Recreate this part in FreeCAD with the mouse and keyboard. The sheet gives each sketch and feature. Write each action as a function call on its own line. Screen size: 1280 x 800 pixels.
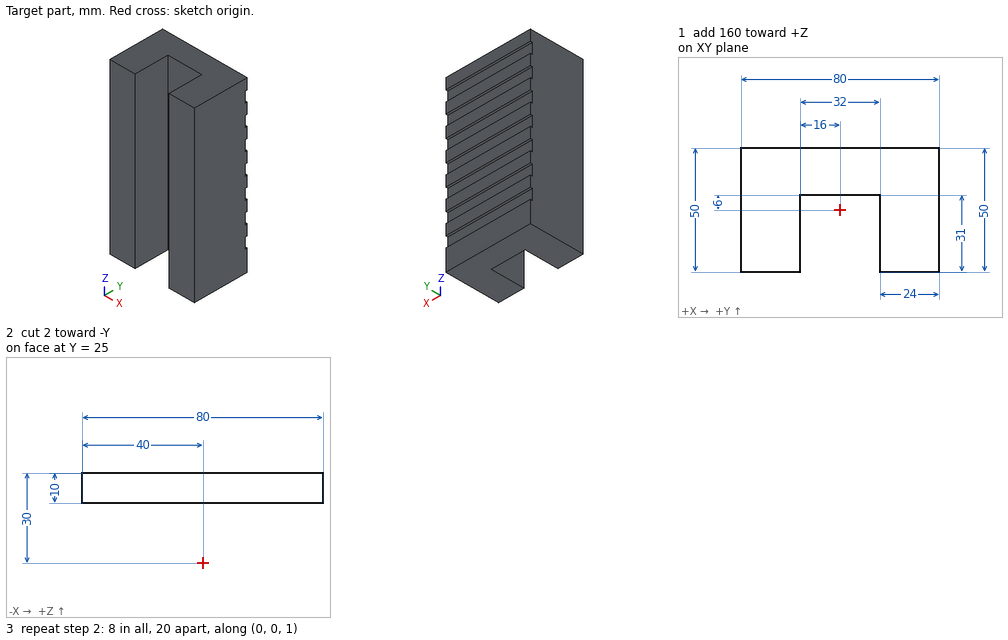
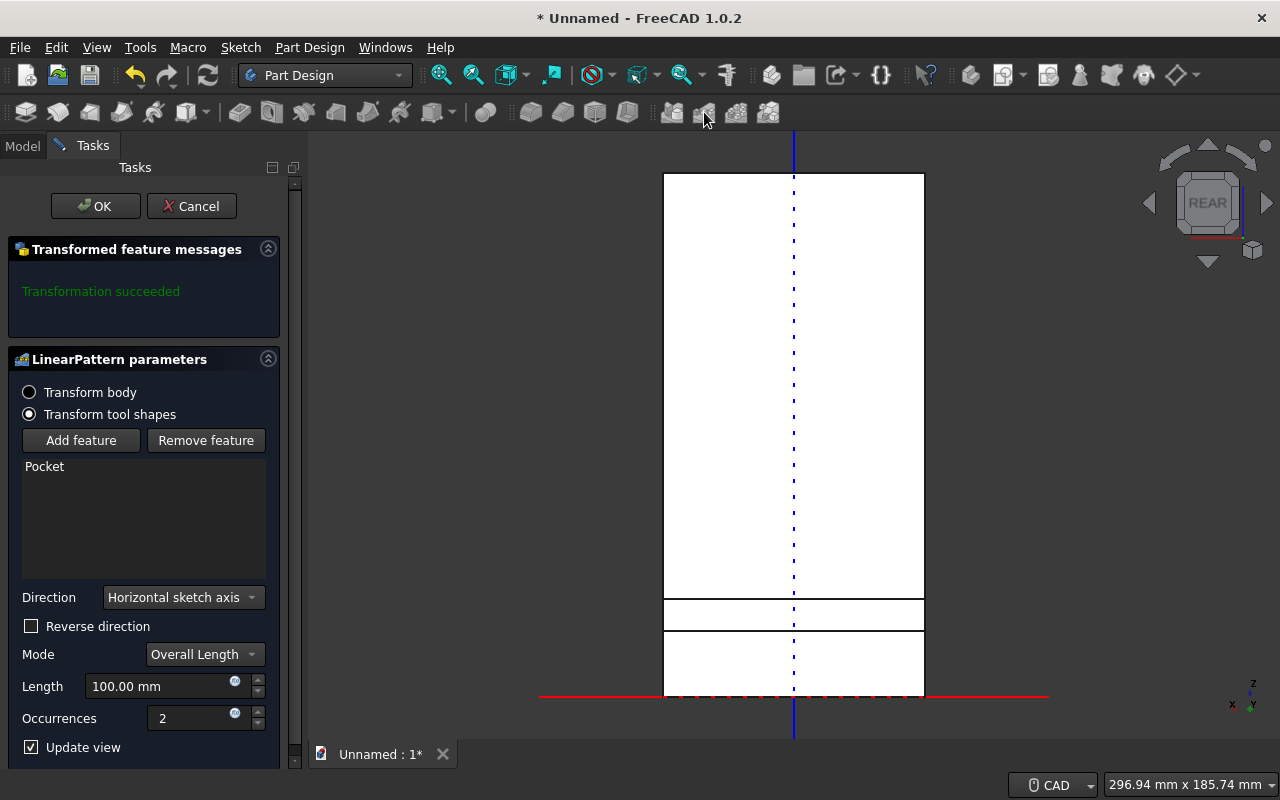
click(184, 598)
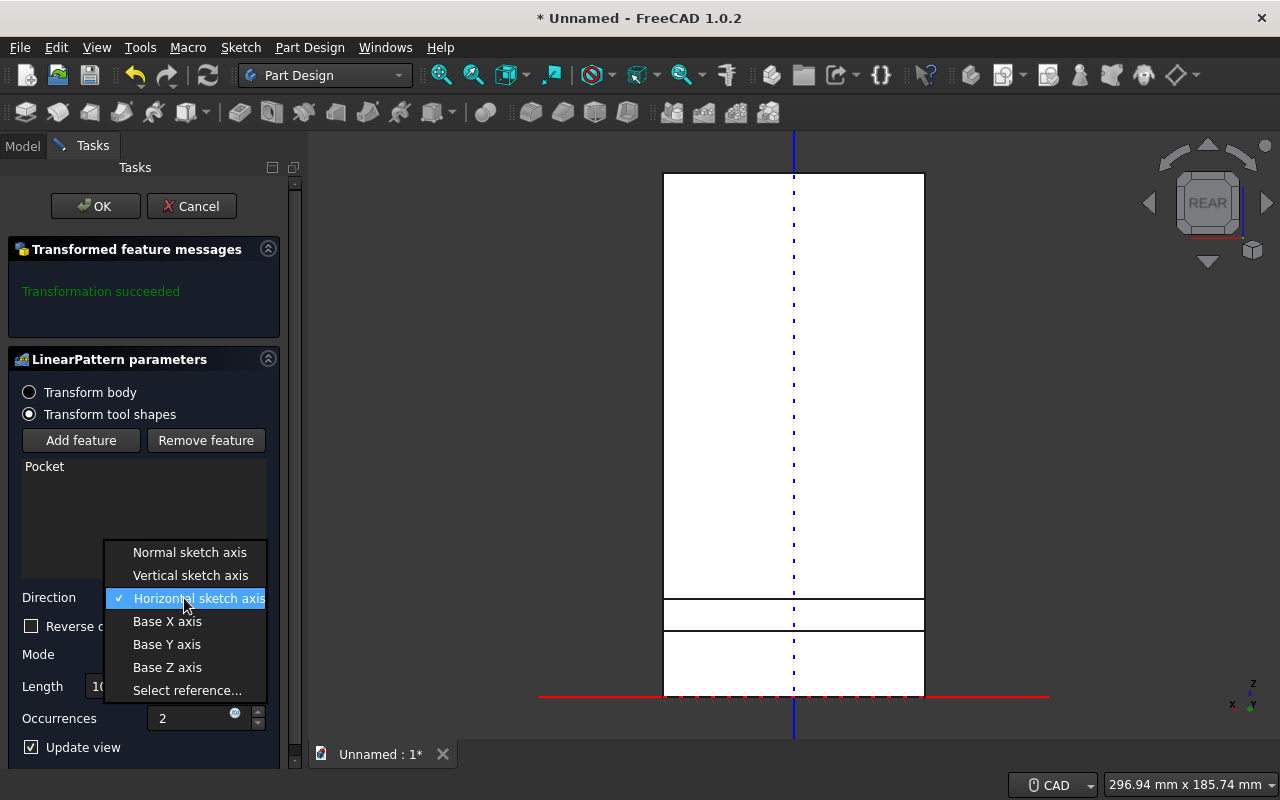
click(184, 668)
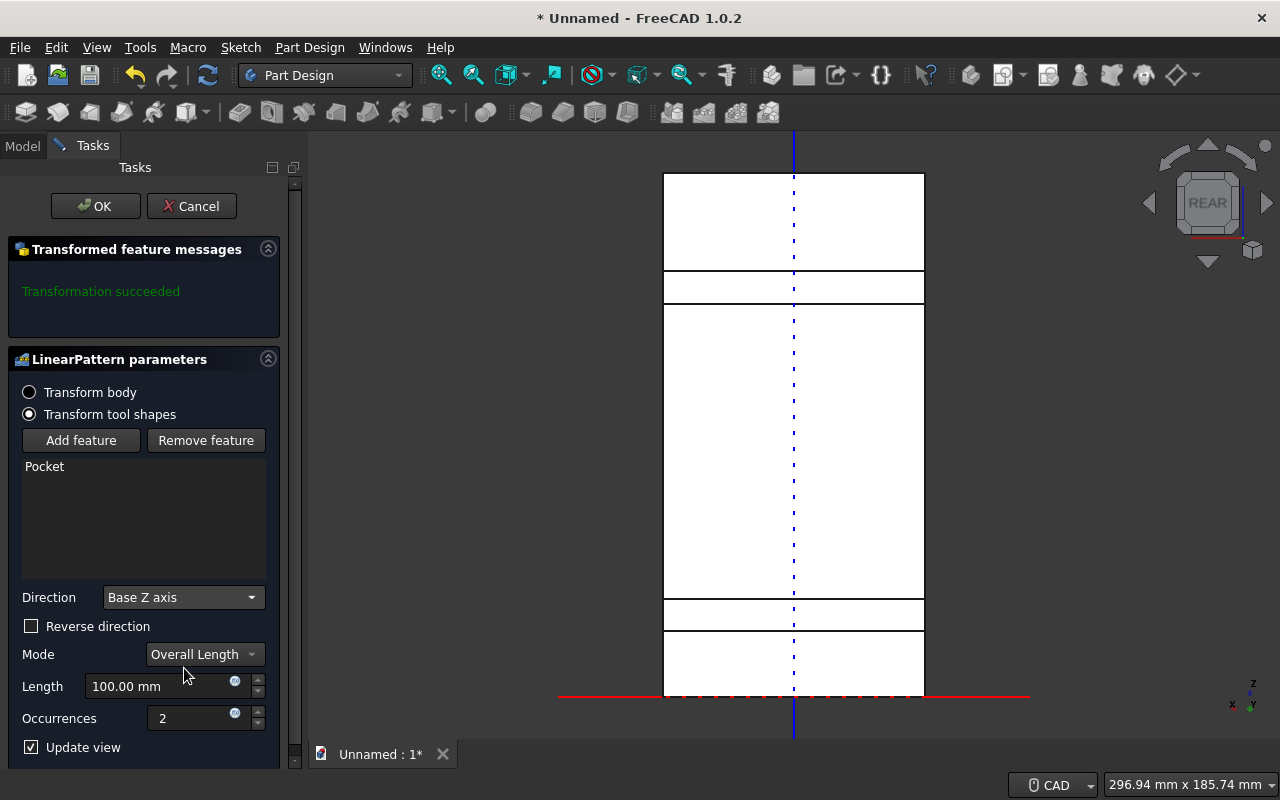
click(206, 654)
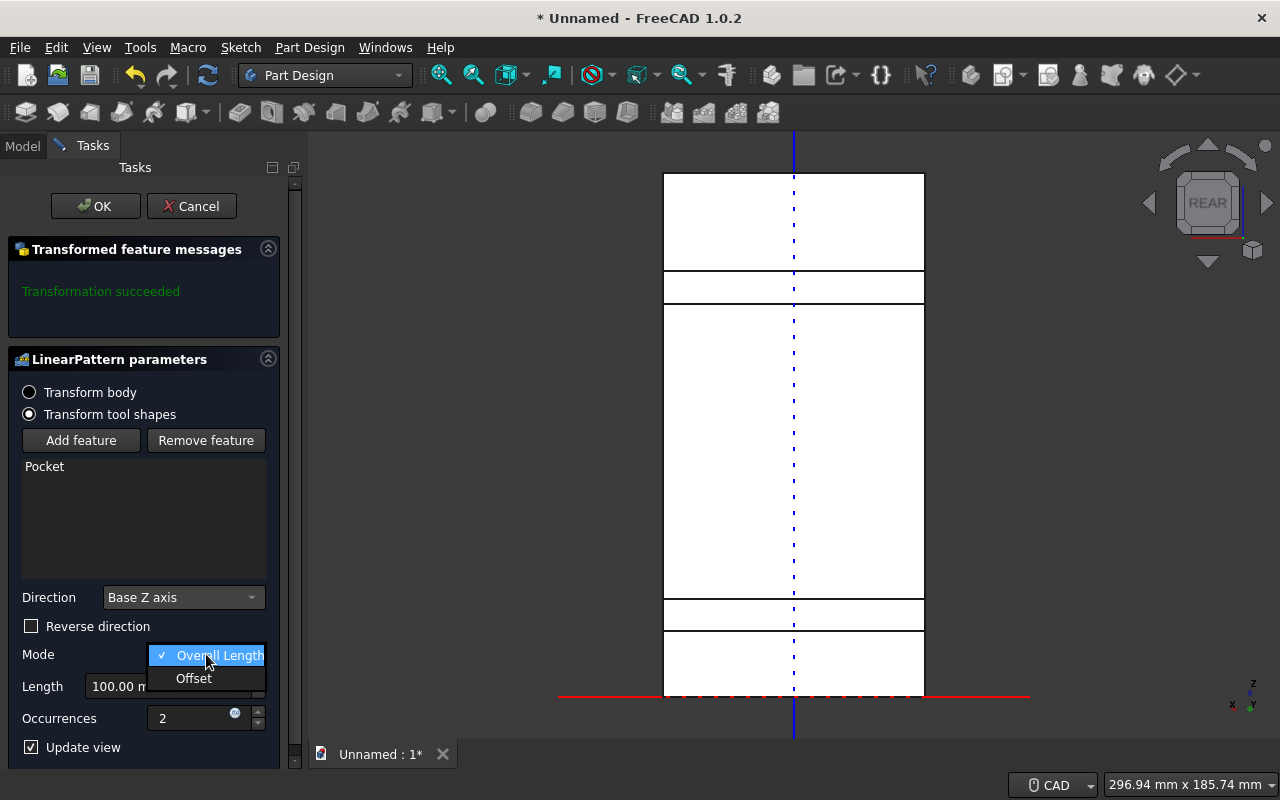
click(206, 678)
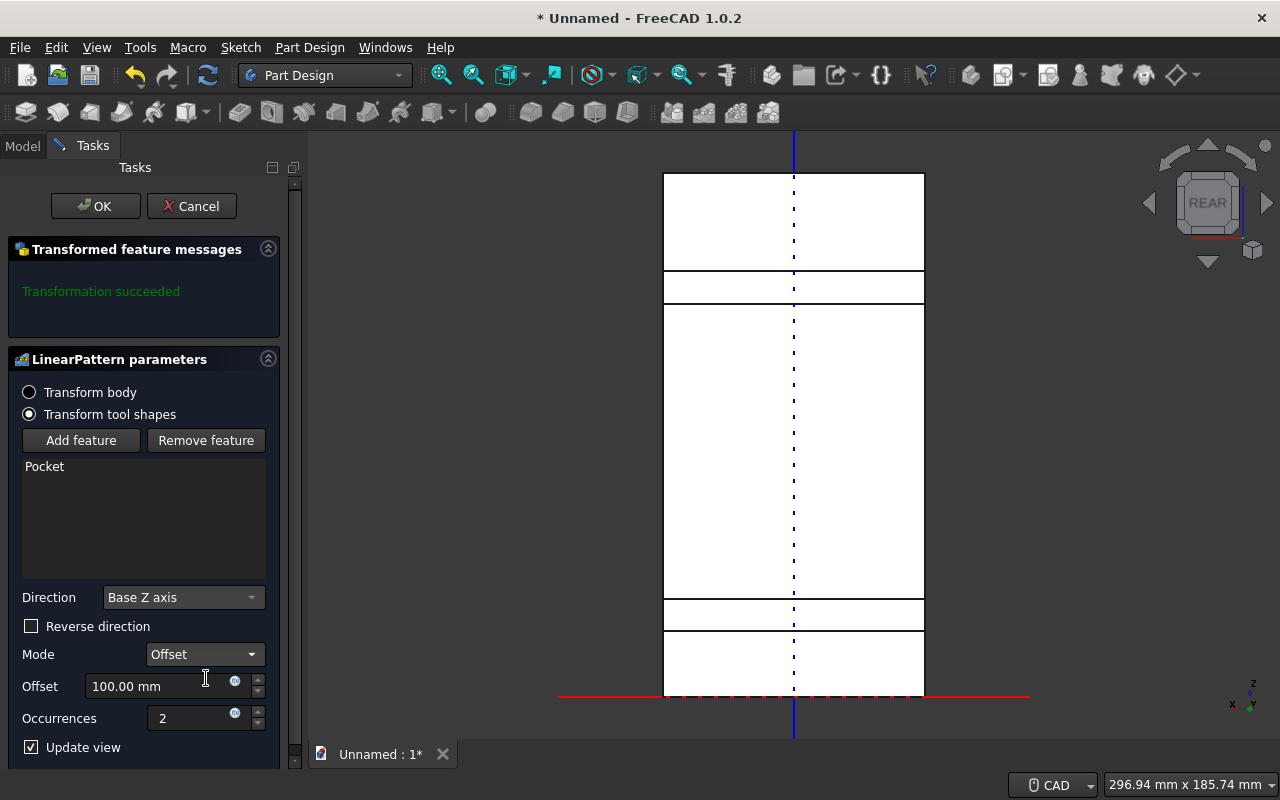
triple_click(168, 686)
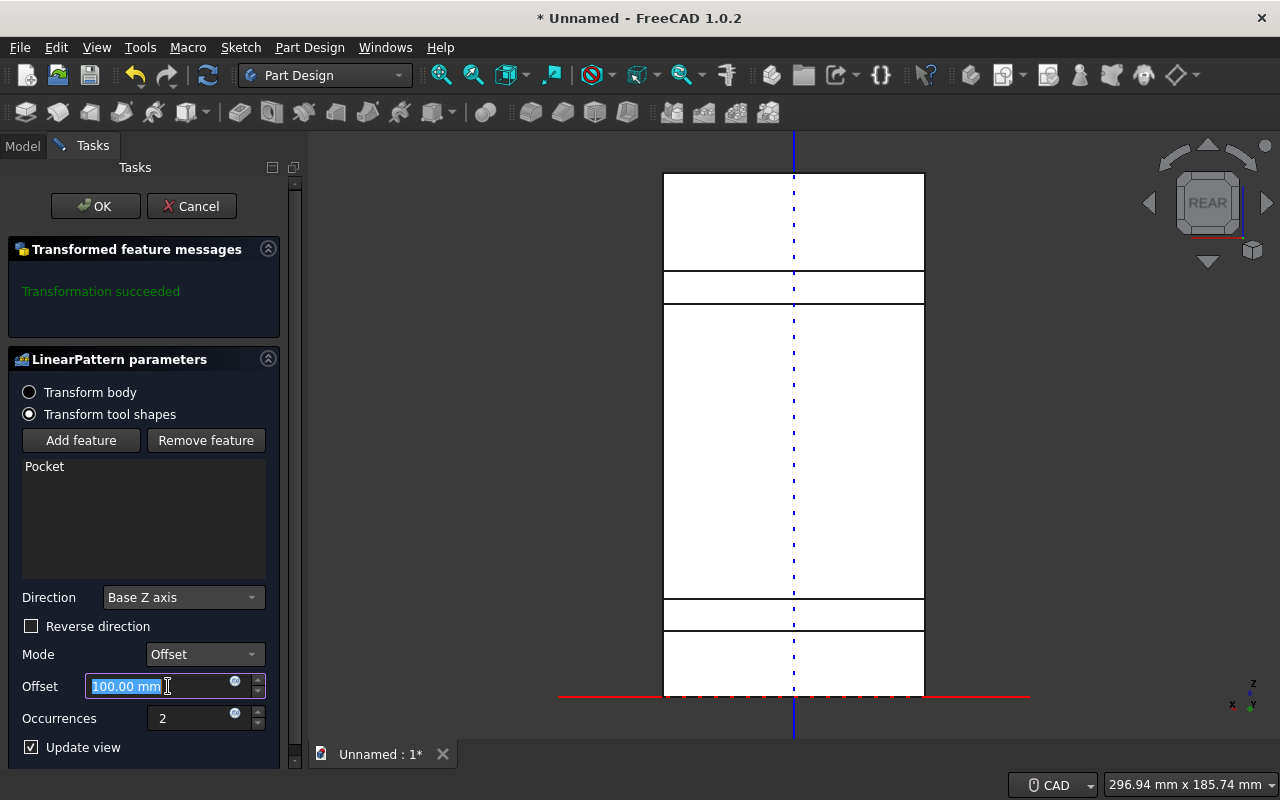
text(20)
key(Tab)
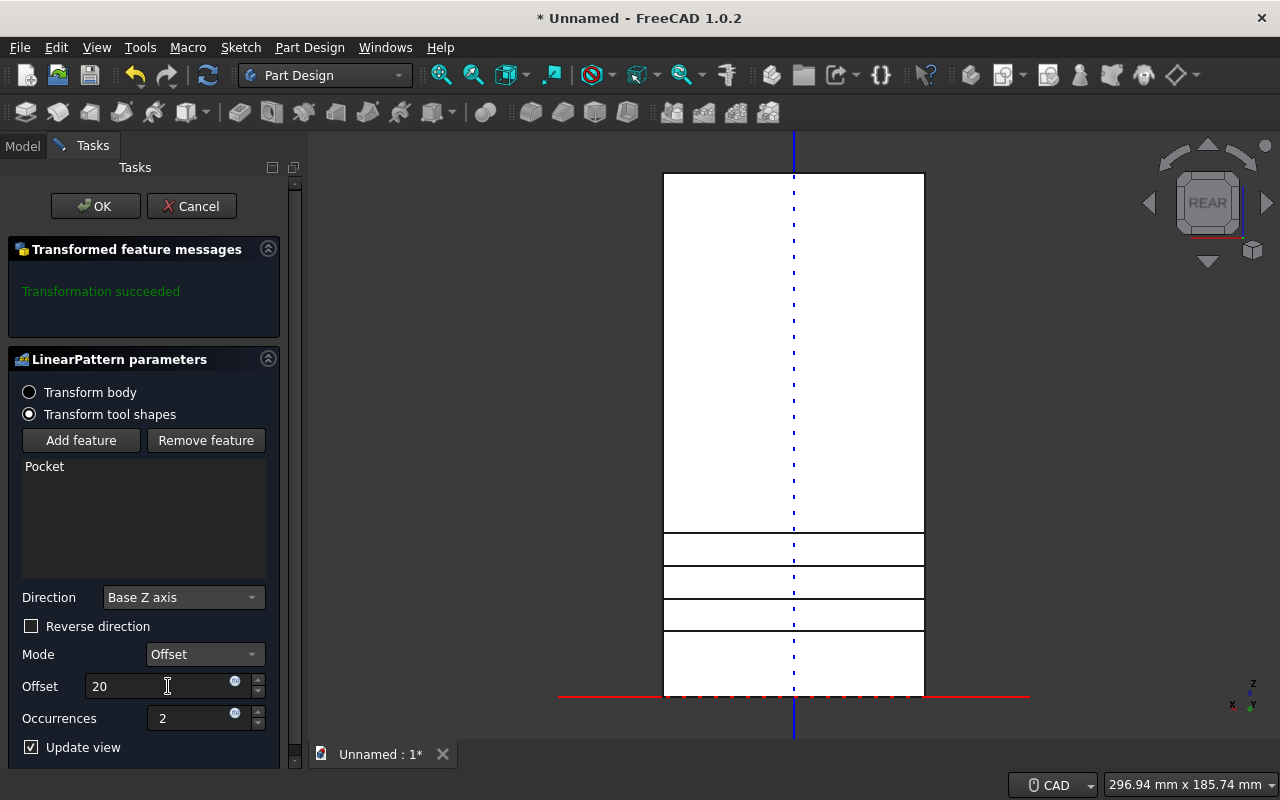
triple_click(198, 718)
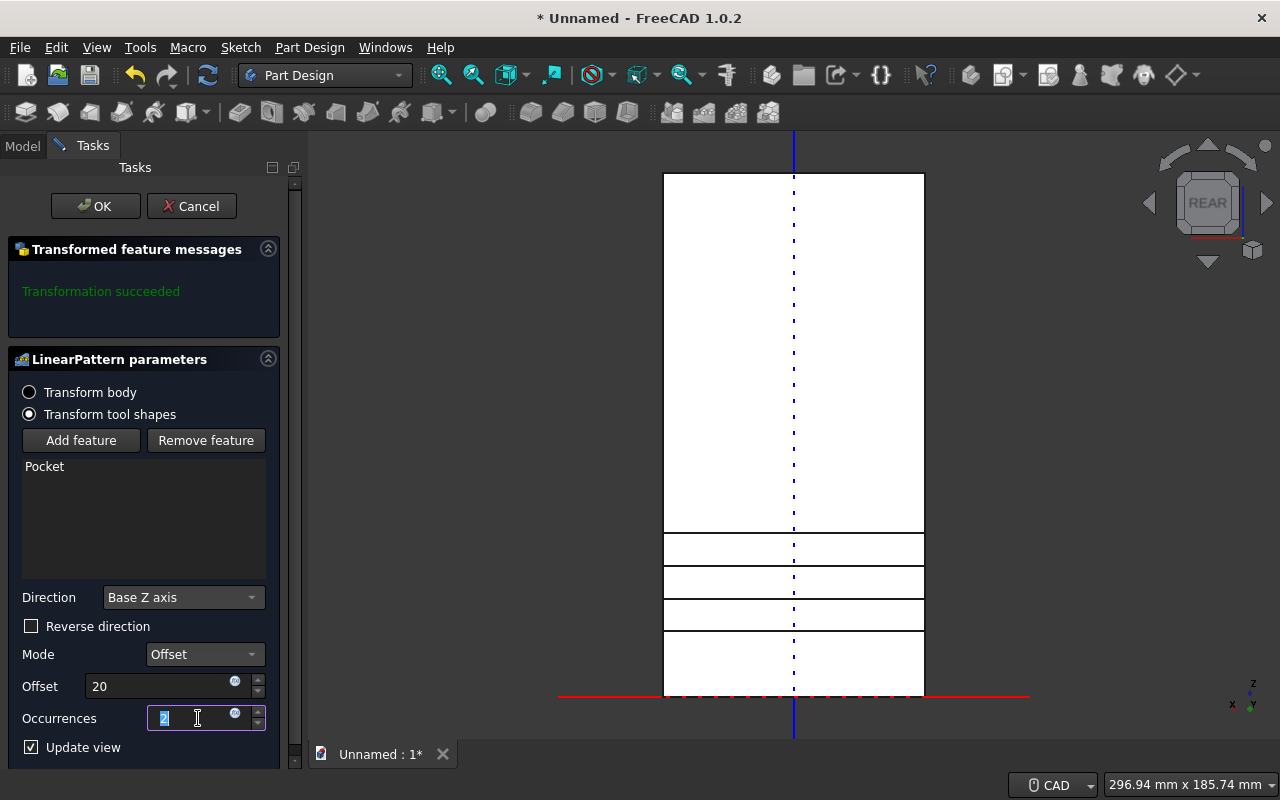
text(8)
key(Tab)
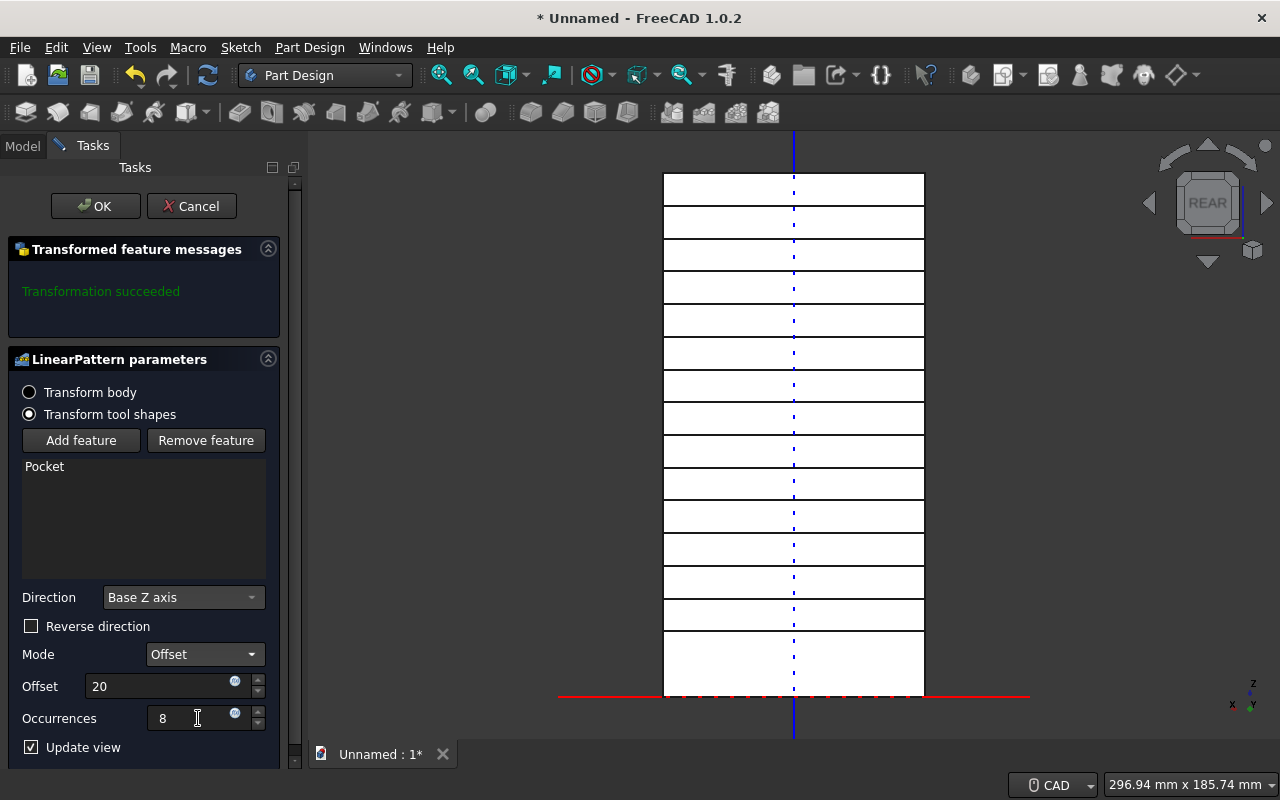
click(96, 206)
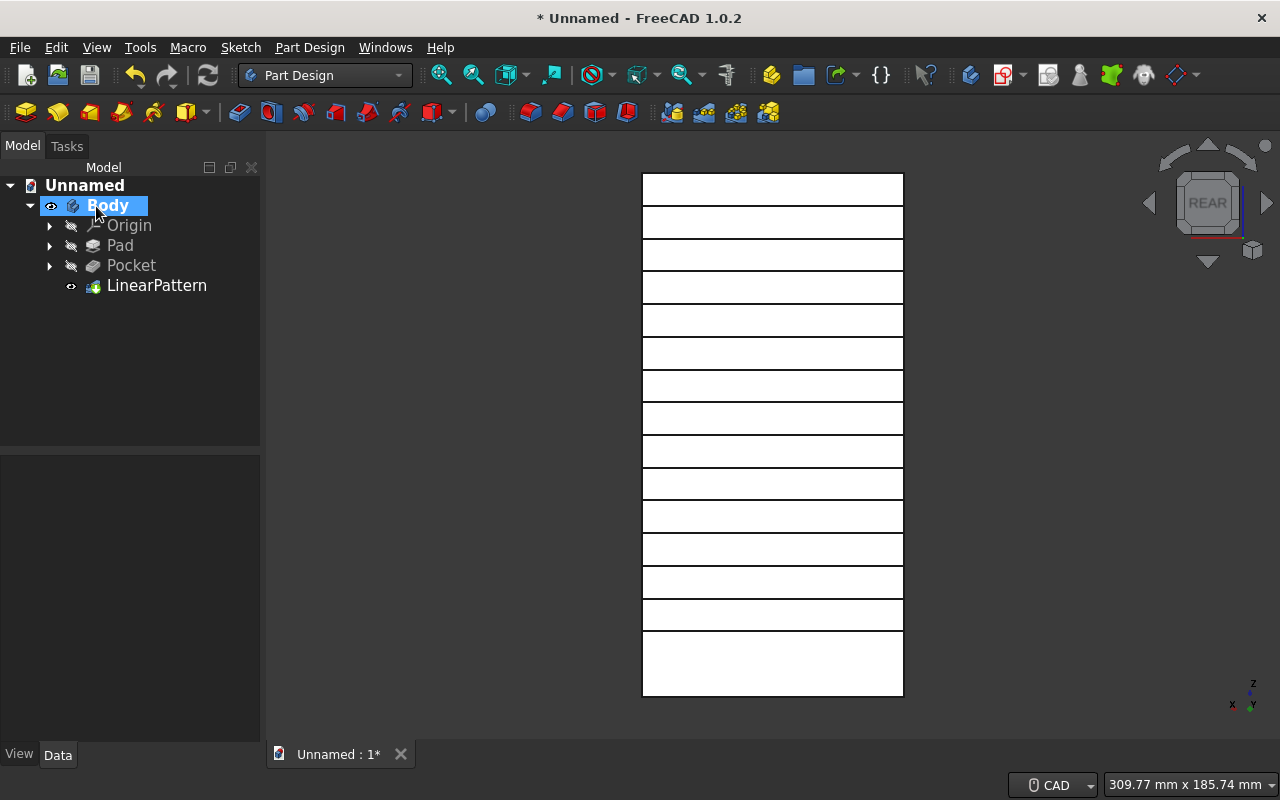
key(0)